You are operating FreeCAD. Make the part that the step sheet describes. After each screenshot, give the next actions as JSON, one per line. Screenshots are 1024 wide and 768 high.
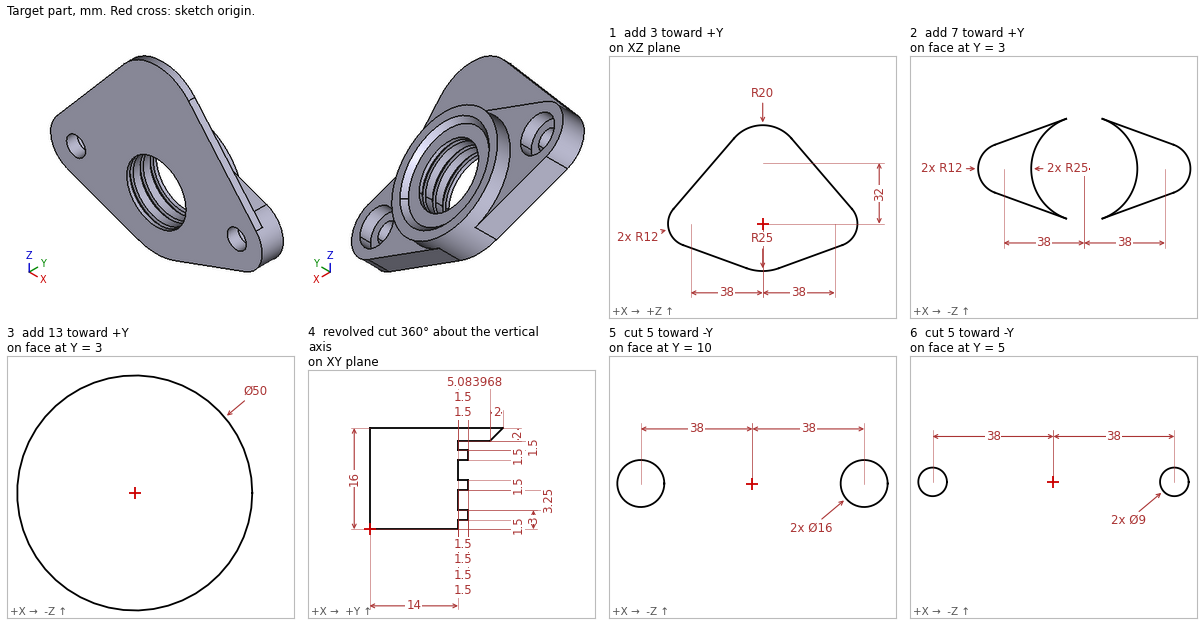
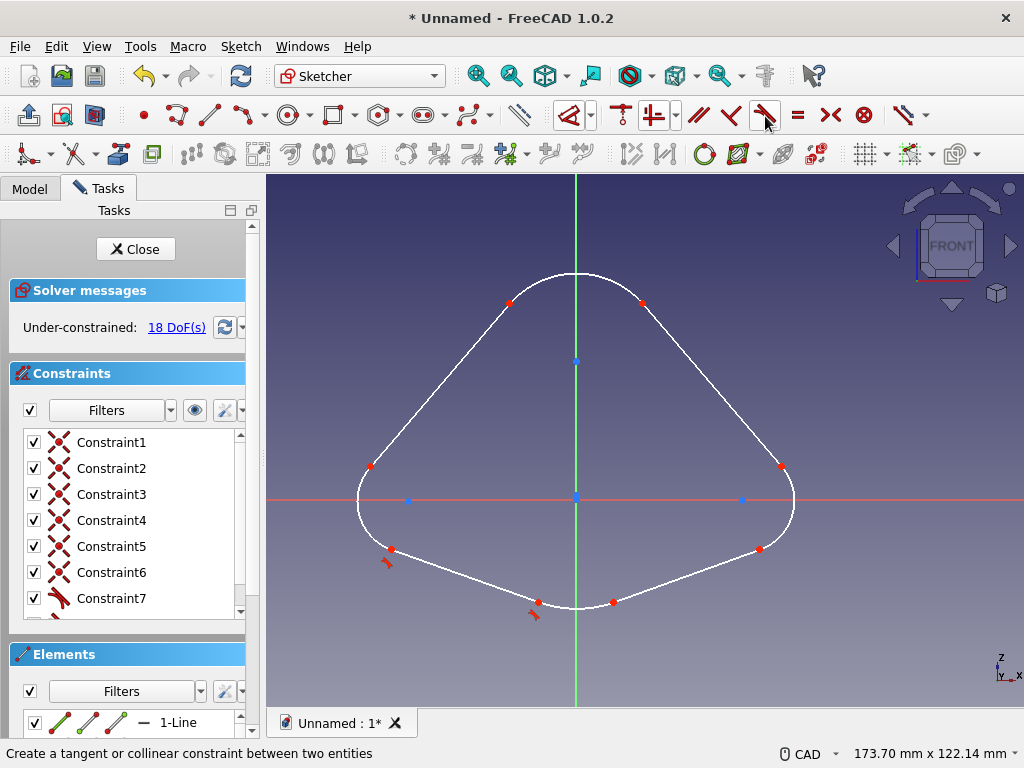
{"action": "left_click", "coordinate": [413, 418]}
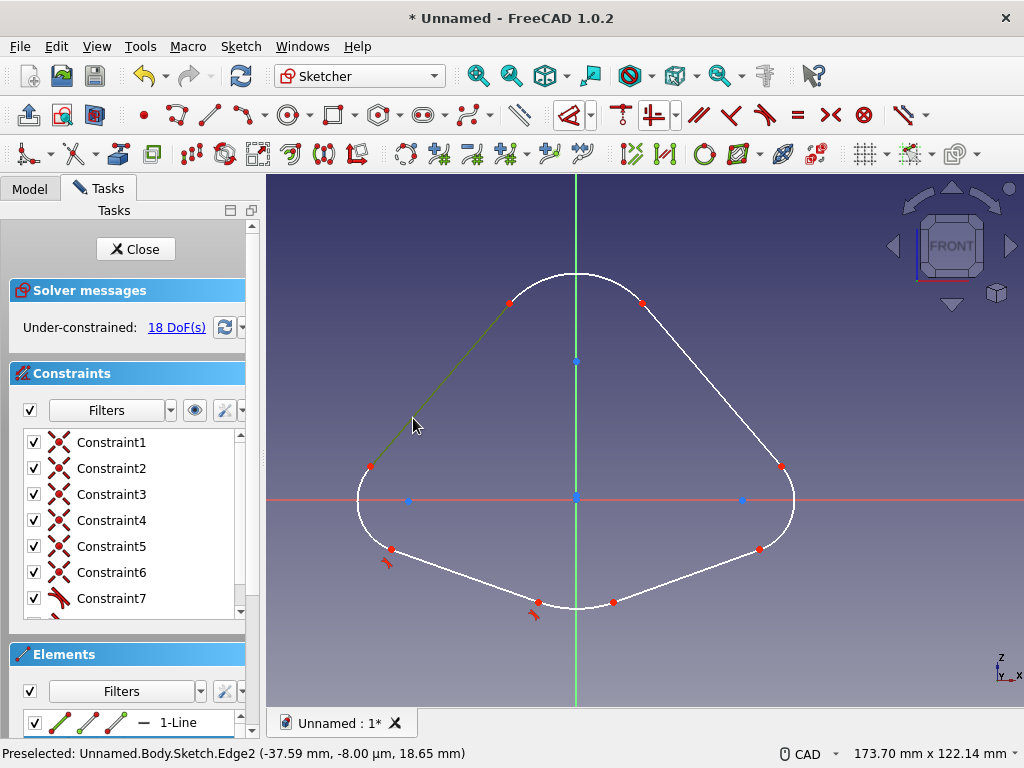
{"action": "left_click", "coordinate": [368, 532]}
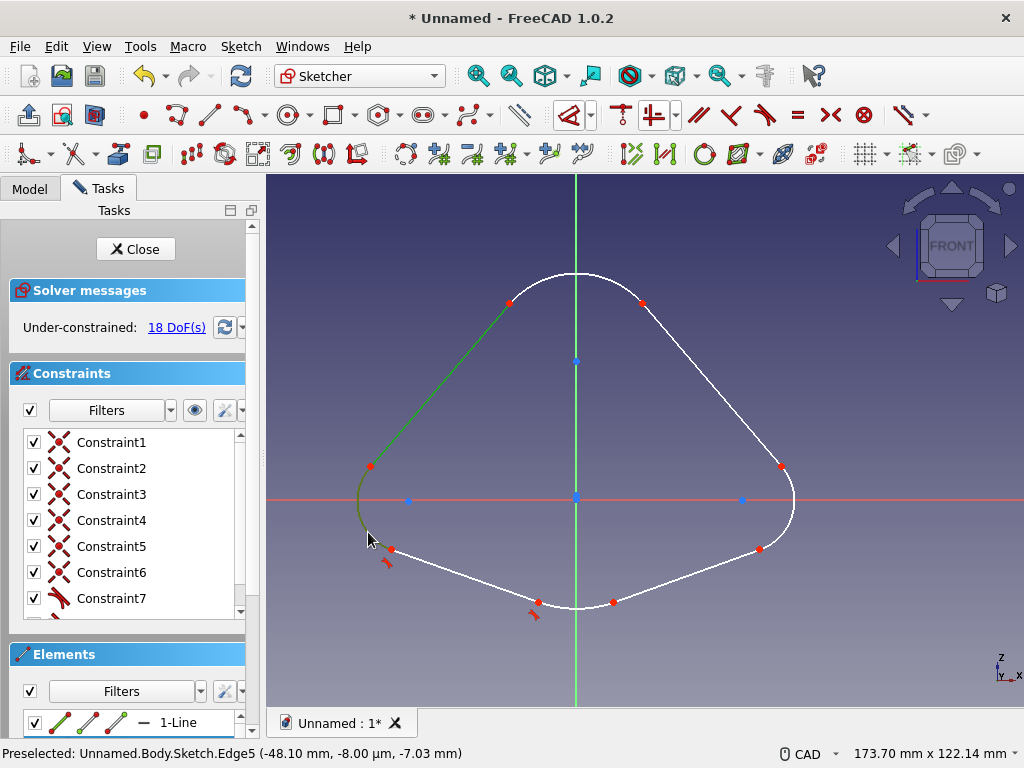
{"action": "left_click", "coordinate": [765, 116]}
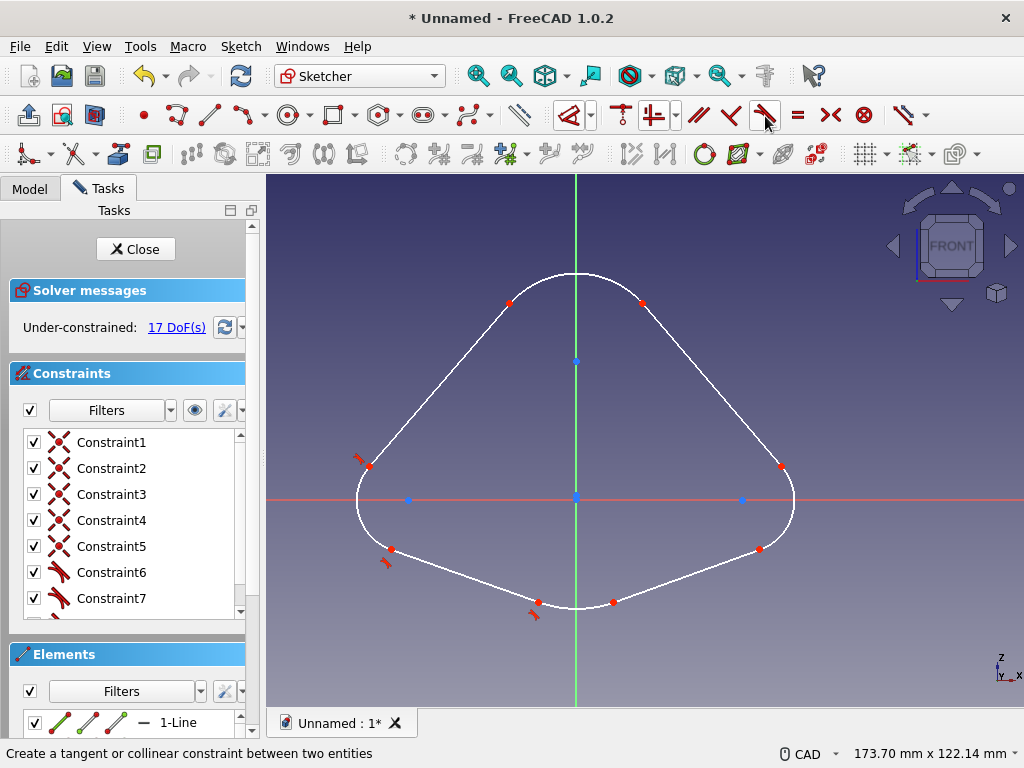
{"action": "left_click", "coordinate": [412, 418]}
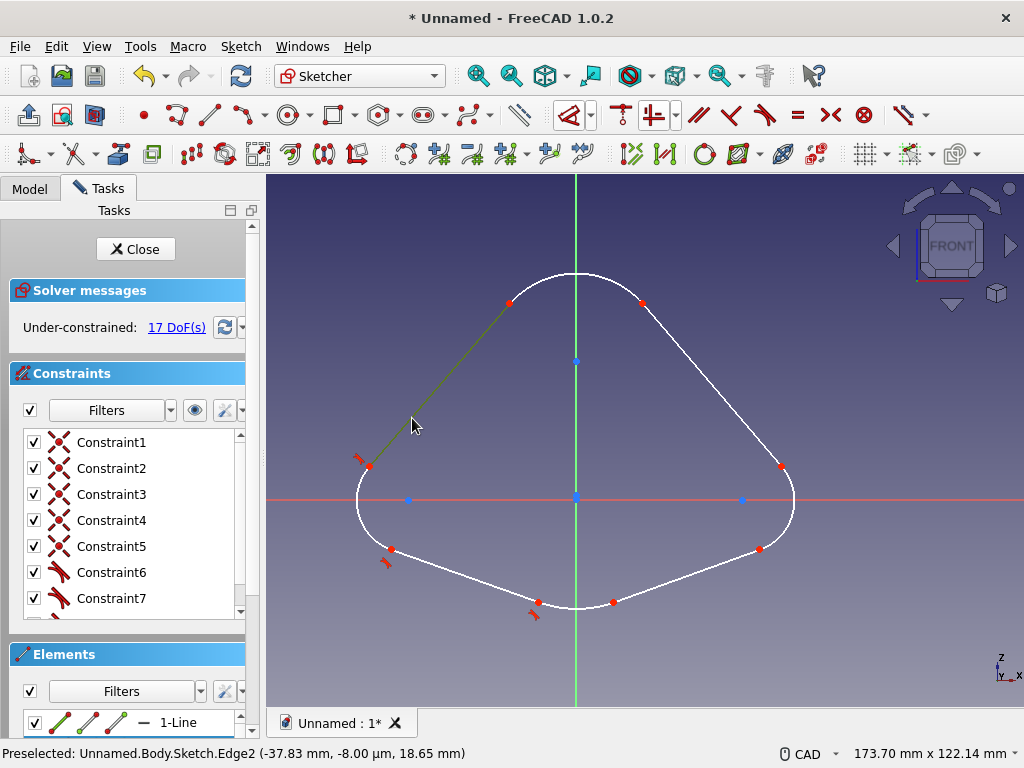
{"action": "left_click", "coordinate": [606, 279]}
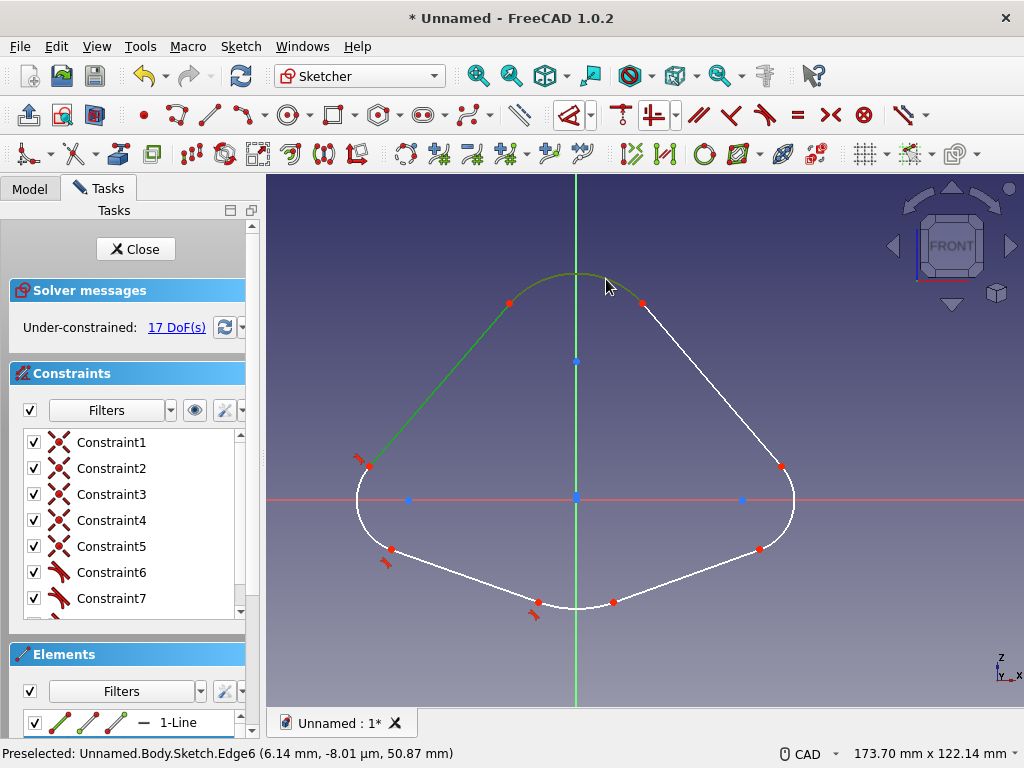
{"action": "left_click", "coordinate": [765, 116]}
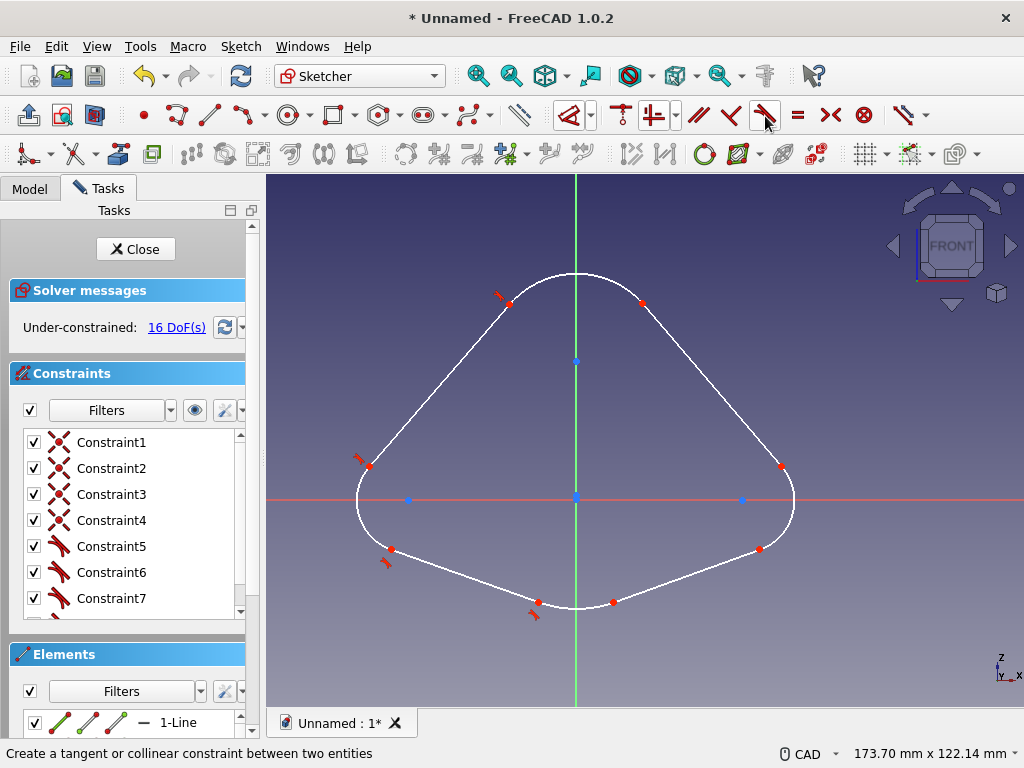
{"action": "left_click", "coordinate": [685, 353]}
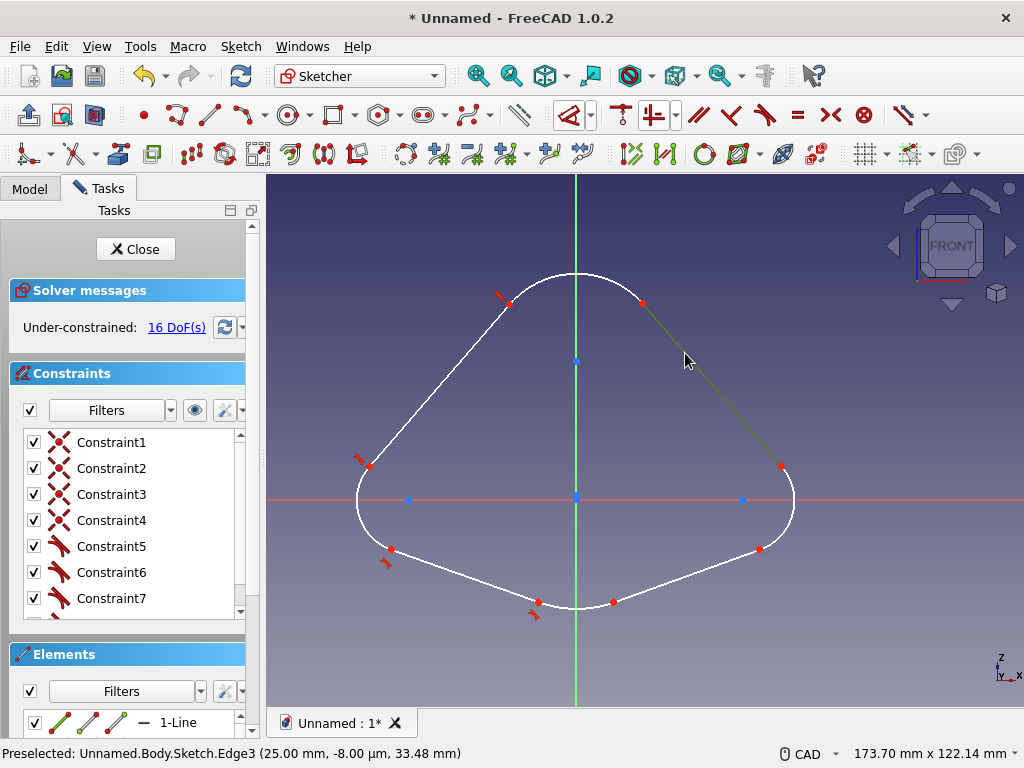
{"action": "left_click", "coordinate": [606, 279]}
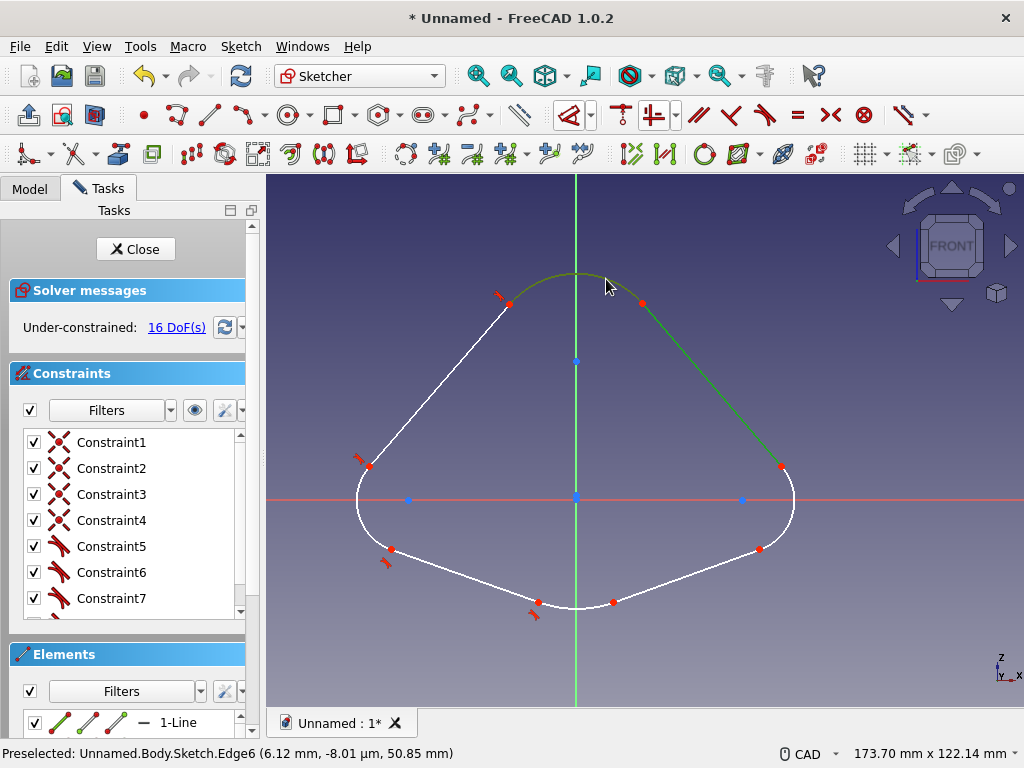
{"action": "left_click", "coordinate": [765, 116]}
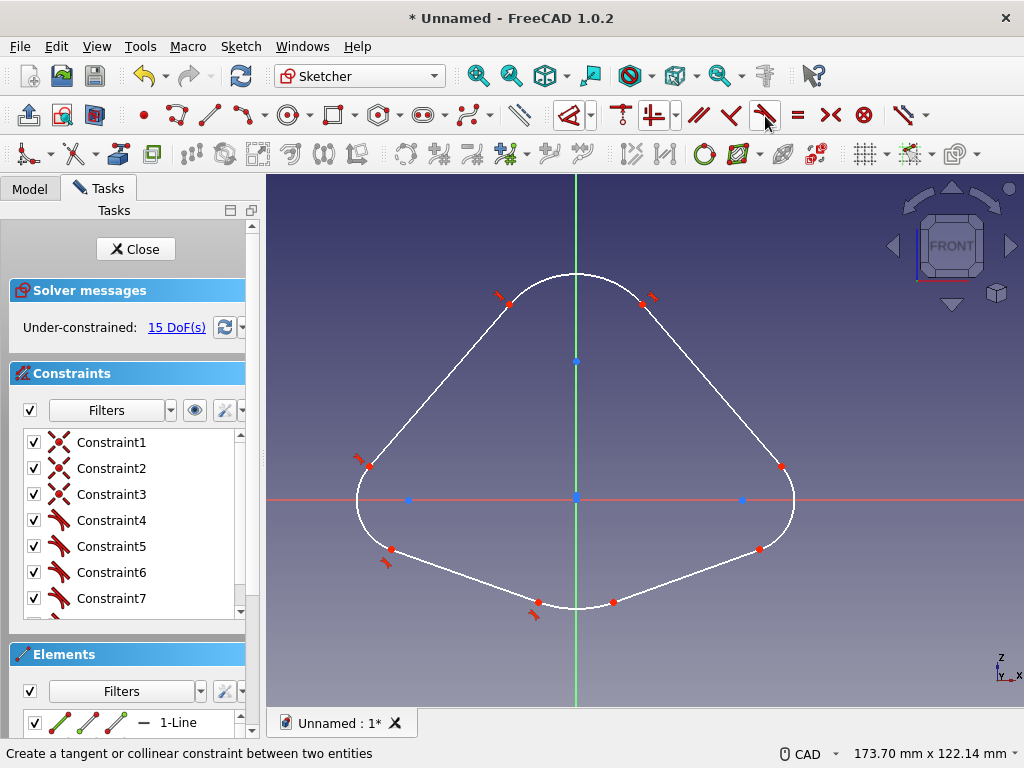
{"action": "left_click", "coordinate": [685, 353]}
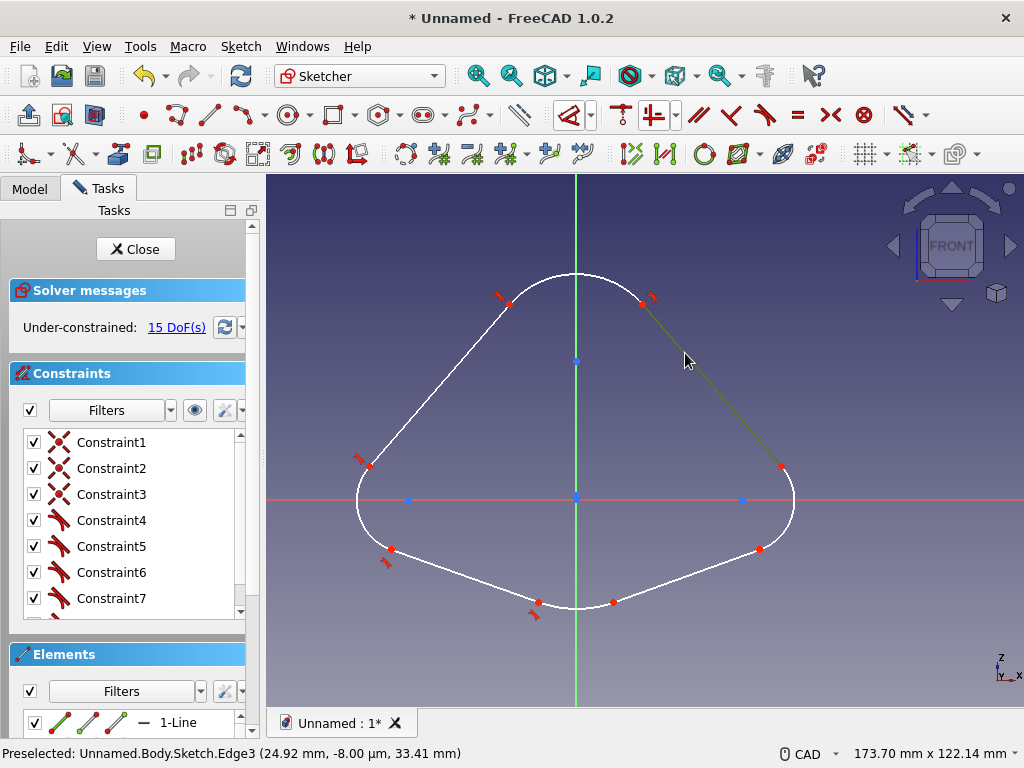
{"action": "left_click", "coordinate": [784, 532]}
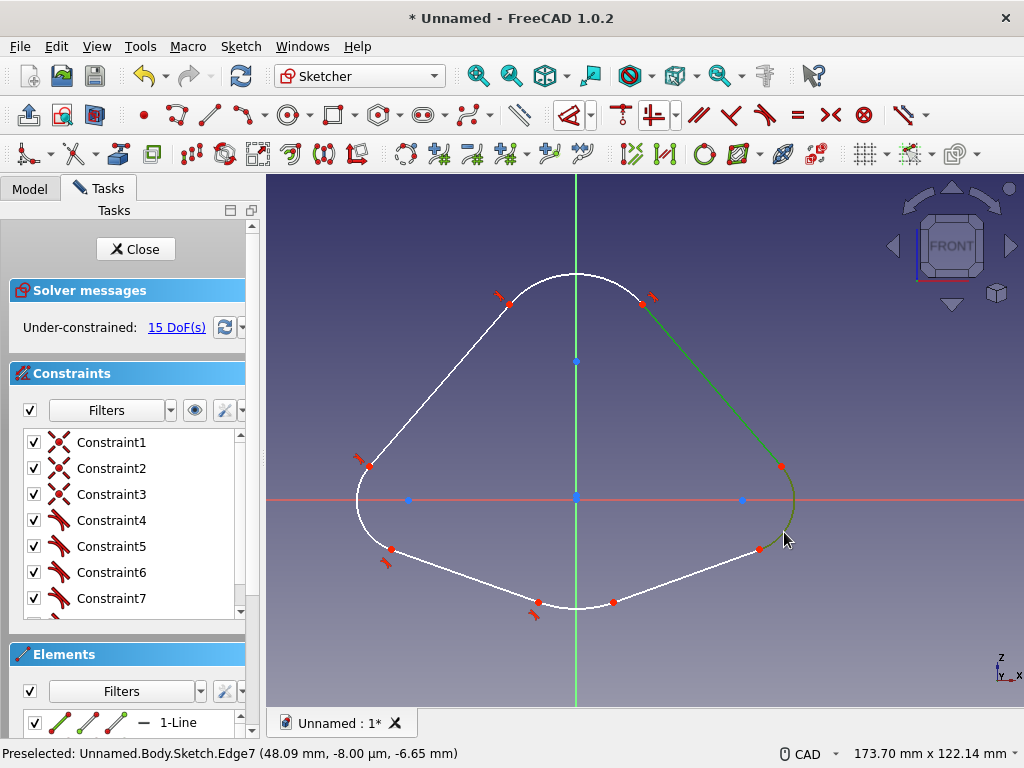
{"action": "left_click", "coordinate": [765, 116]}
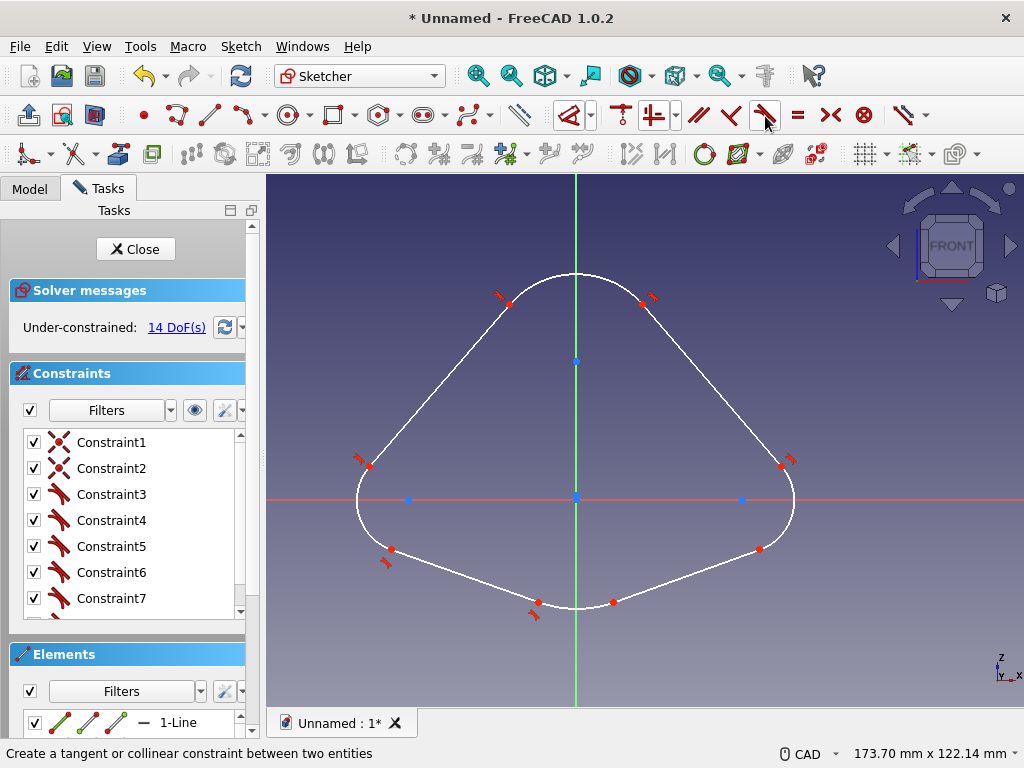
{"action": "left_click", "coordinate": [716, 566]}